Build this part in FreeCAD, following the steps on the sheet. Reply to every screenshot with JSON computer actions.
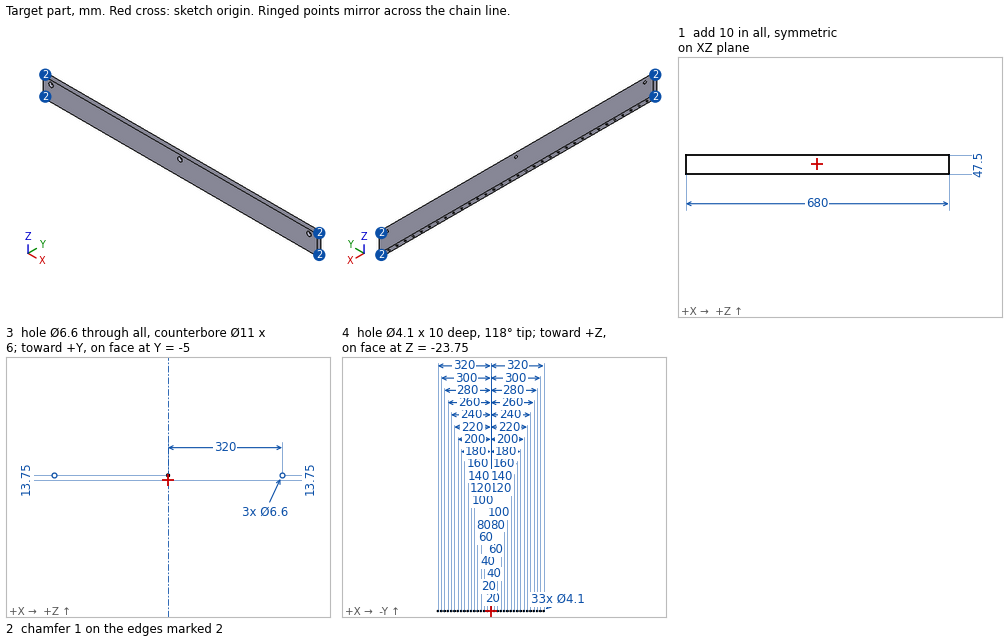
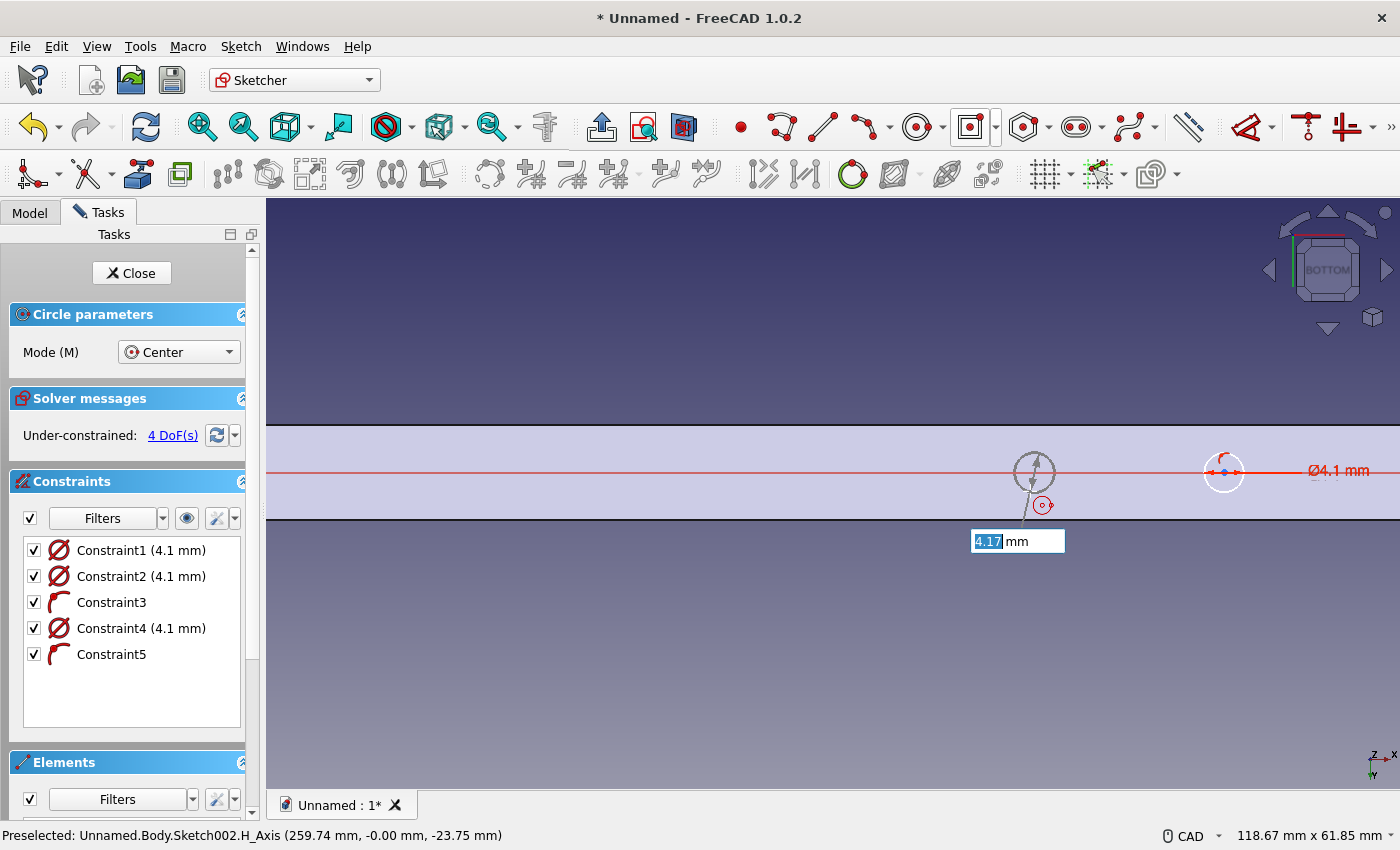
{"action": "type", "text": "4.1"}
{"action": "key", "text": "Return"}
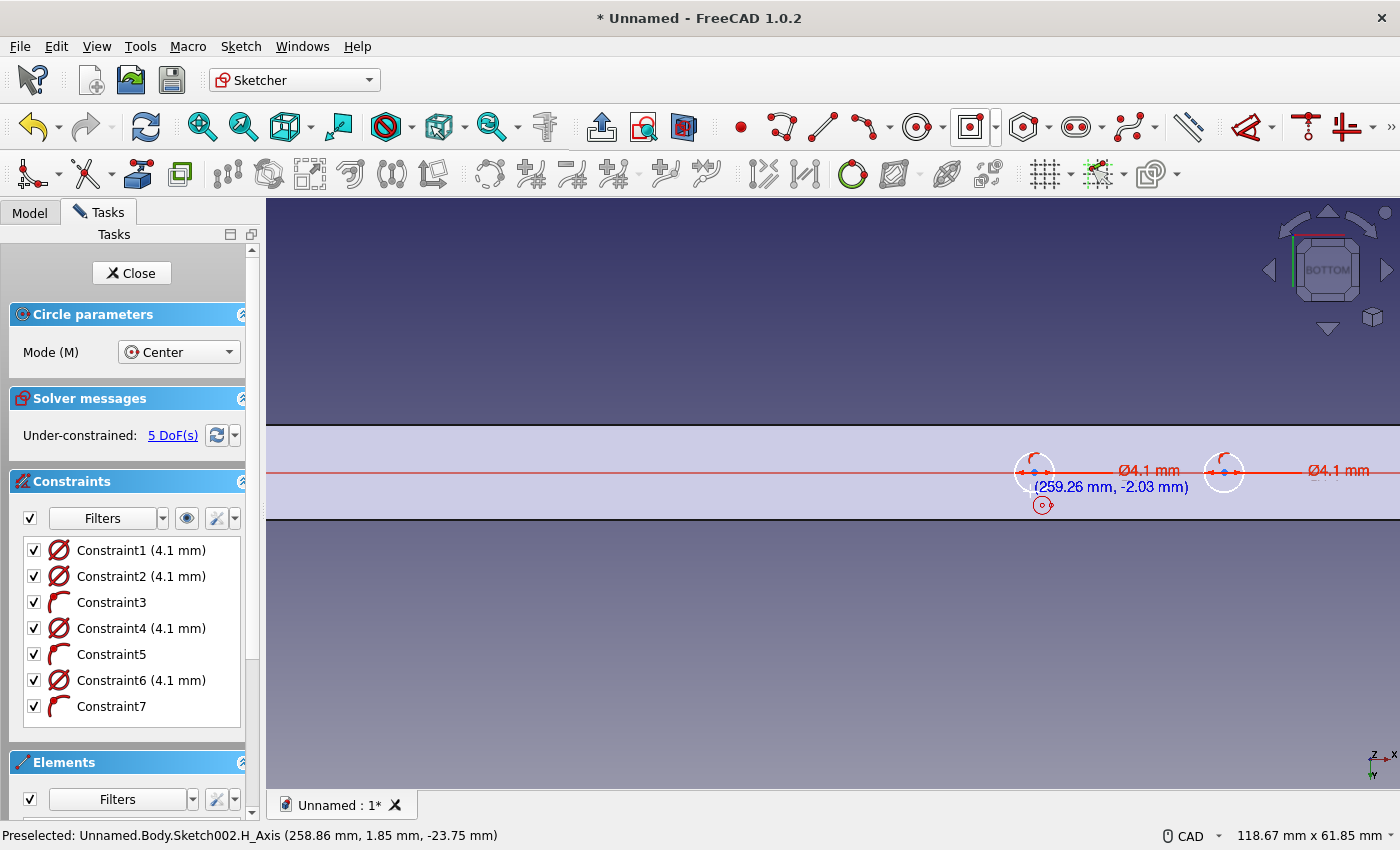
{"action": "scroll", "coordinate": [1040, 496], "scroll_direction": "down", "scroll_amount": 11}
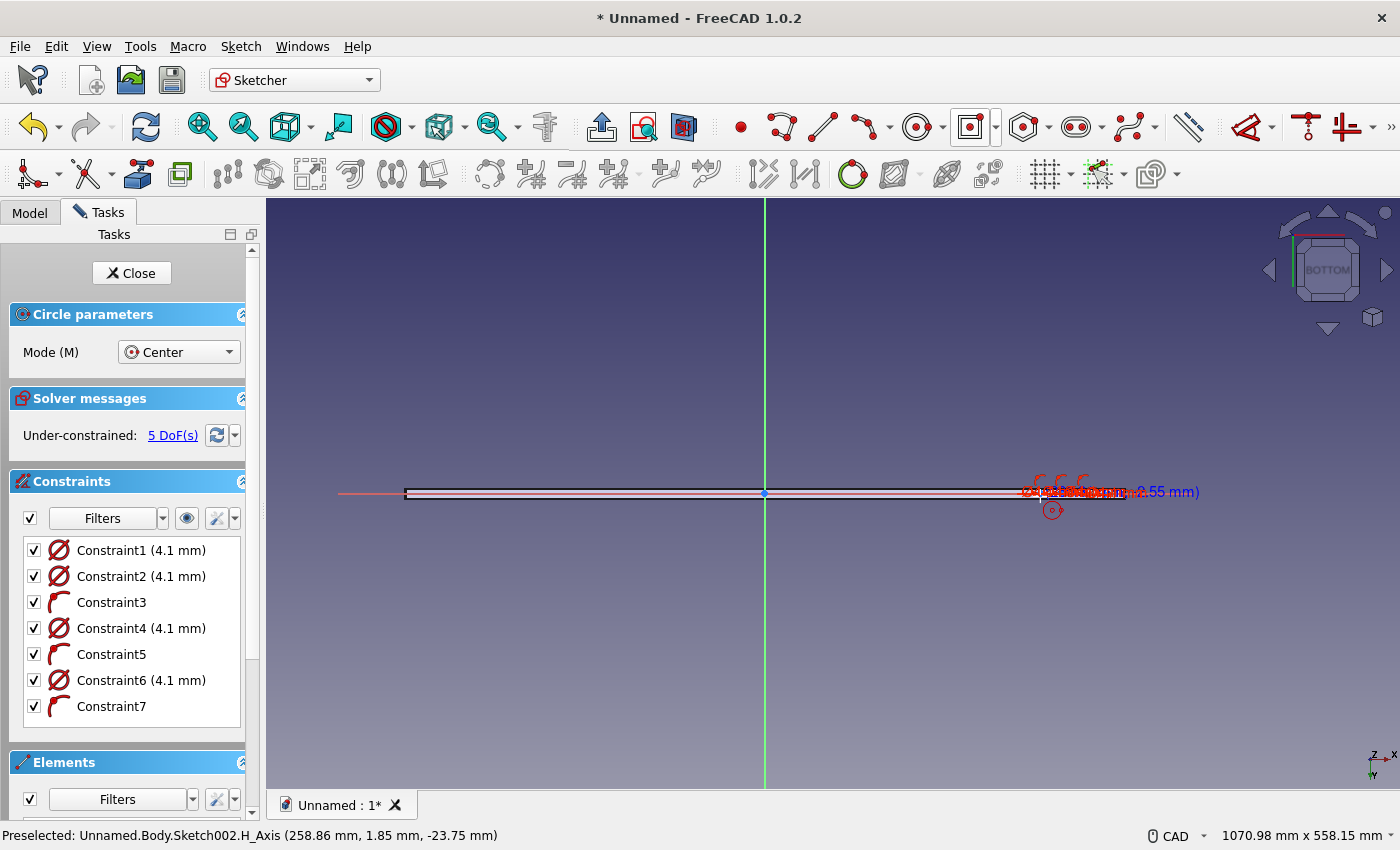
{"action": "left_click", "coordinate": [1019, 494]}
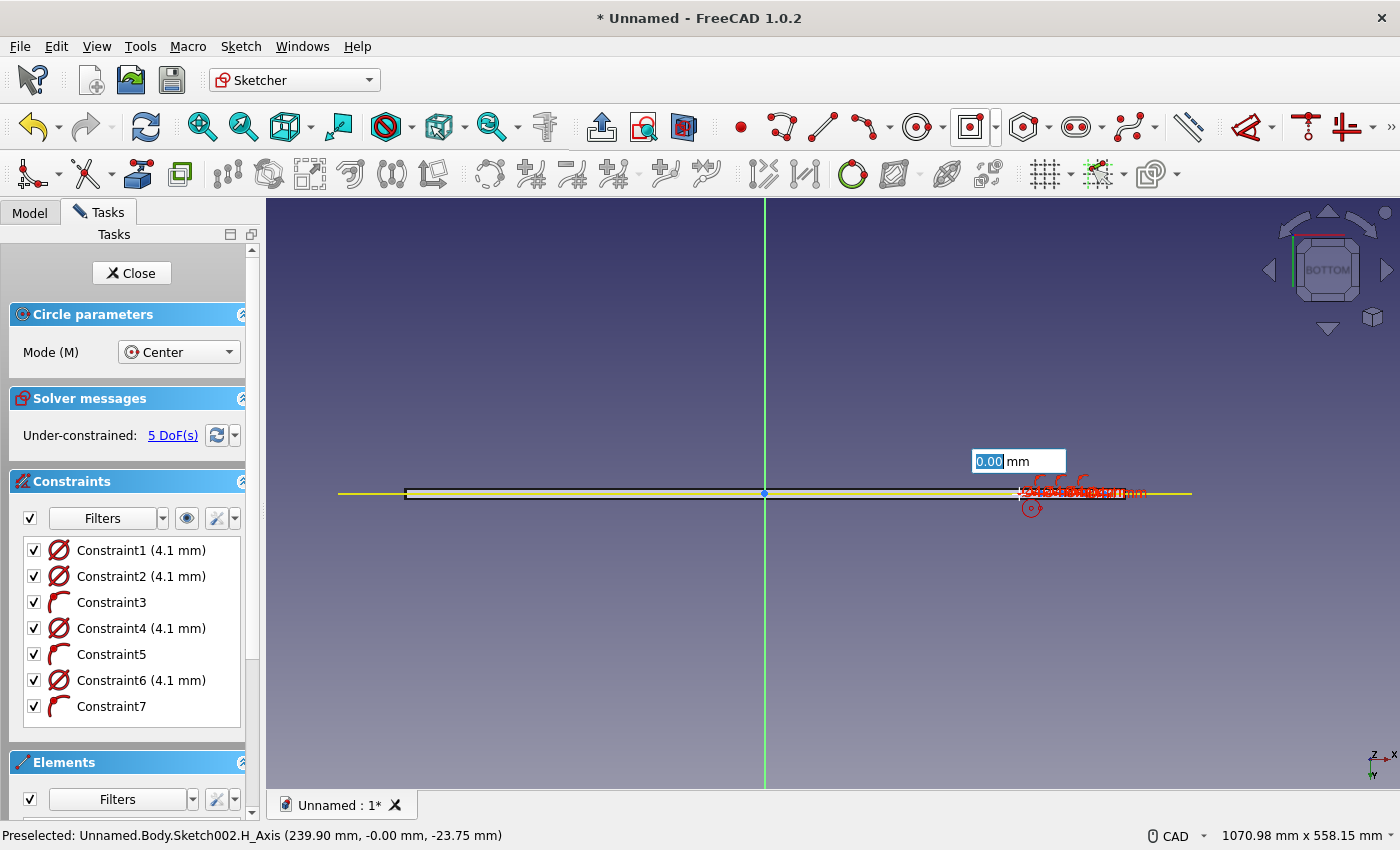
{"action": "scroll", "coordinate": [1018, 496], "scroll_direction": "up", "scroll_amount": 11}
{"action": "mouse_move", "coordinate": [1016, 491]}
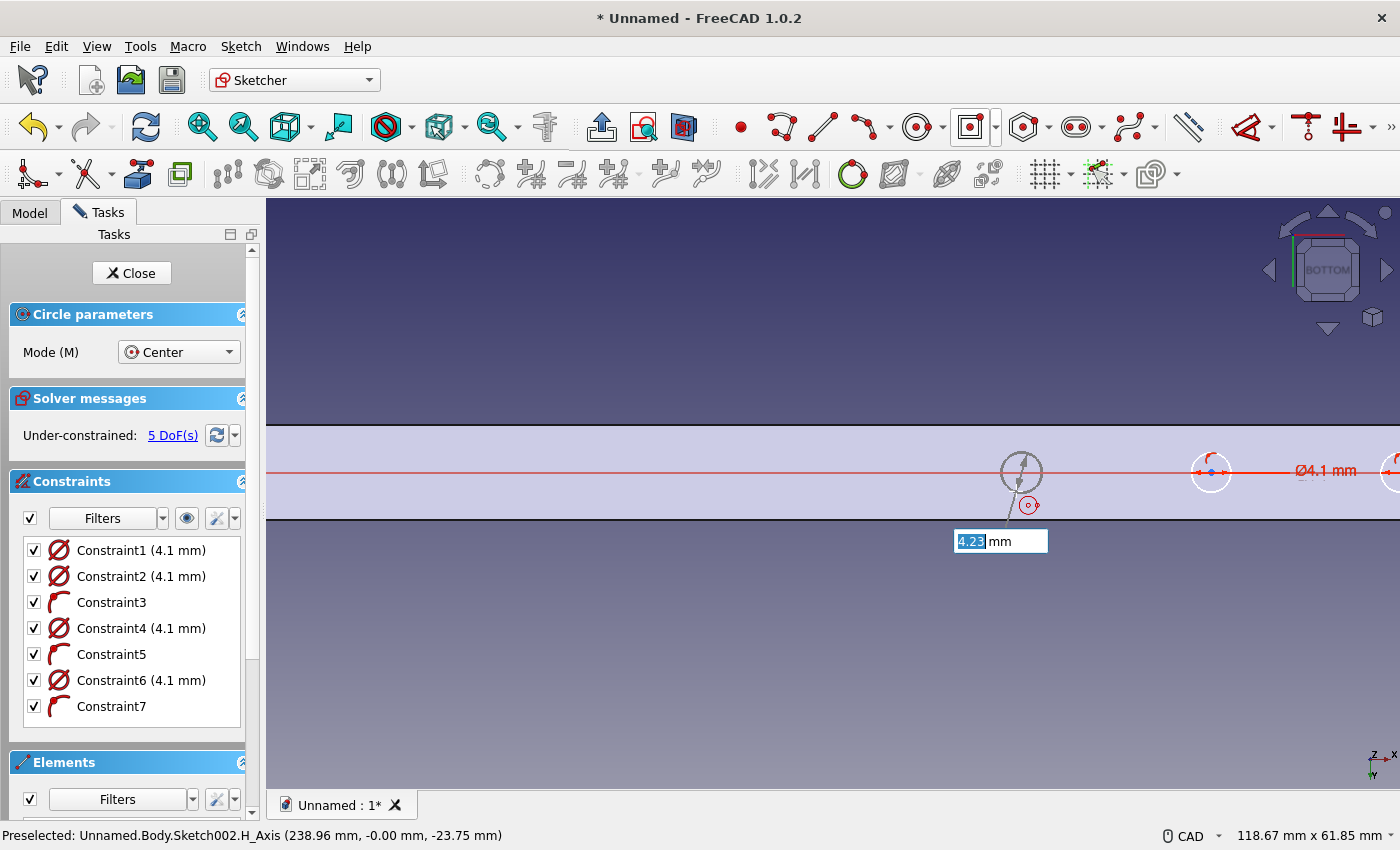
{"action": "type", "text": "4.1"}
{"action": "key", "text": "Return"}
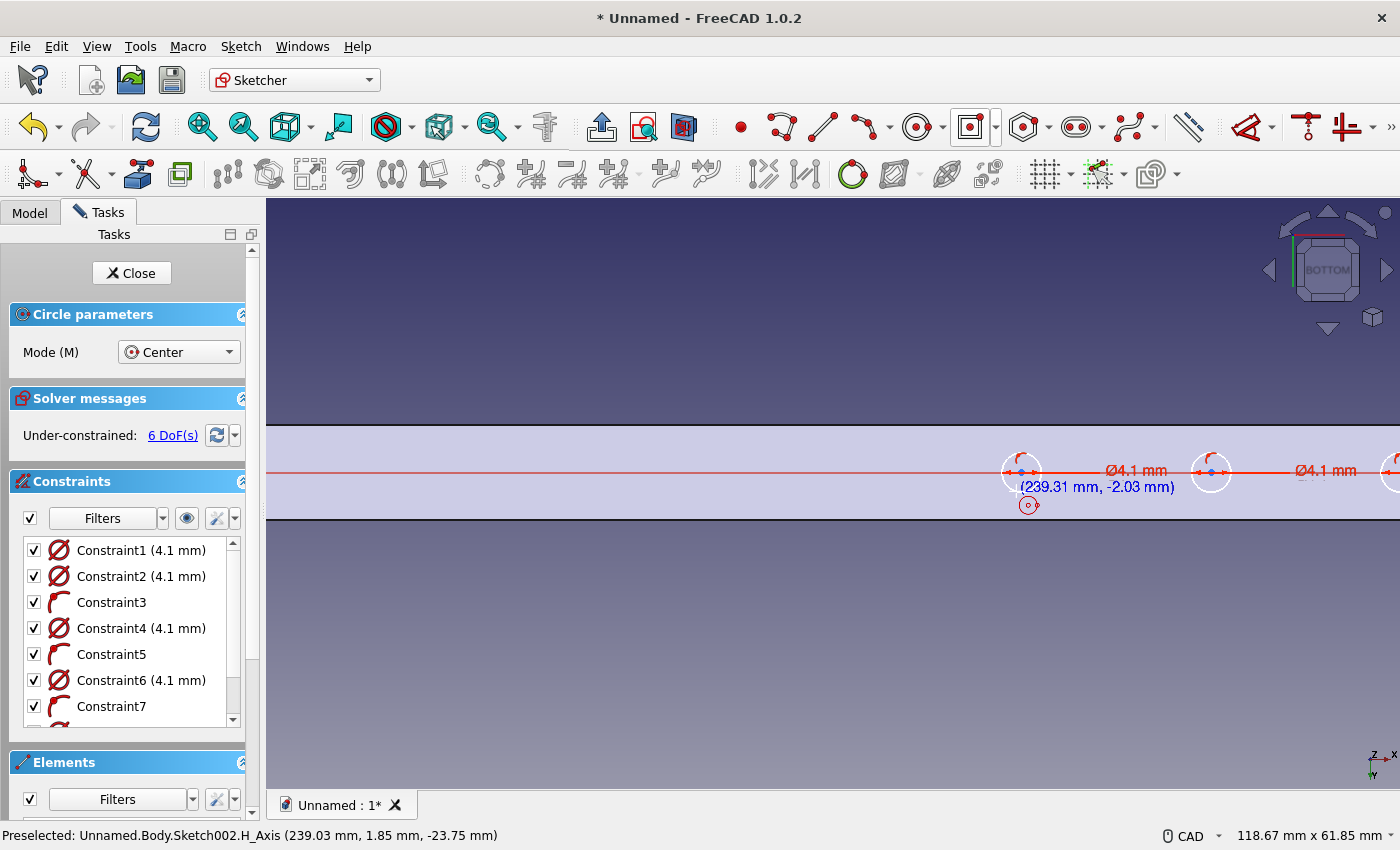
{"action": "scroll", "coordinate": [1018, 496], "scroll_direction": "down", "scroll_amount": 11}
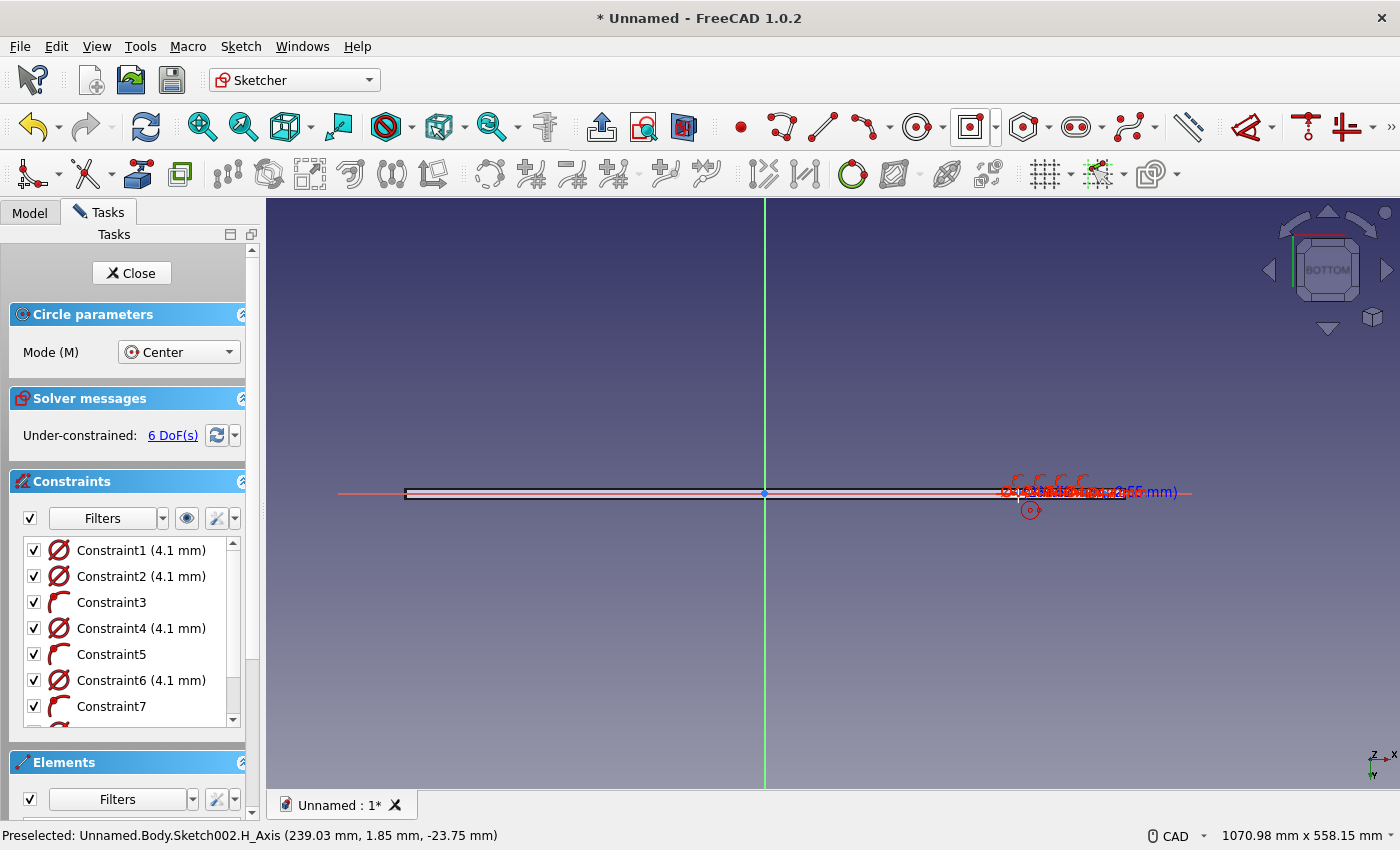
{"action": "left_click", "coordinate": [998, 494]}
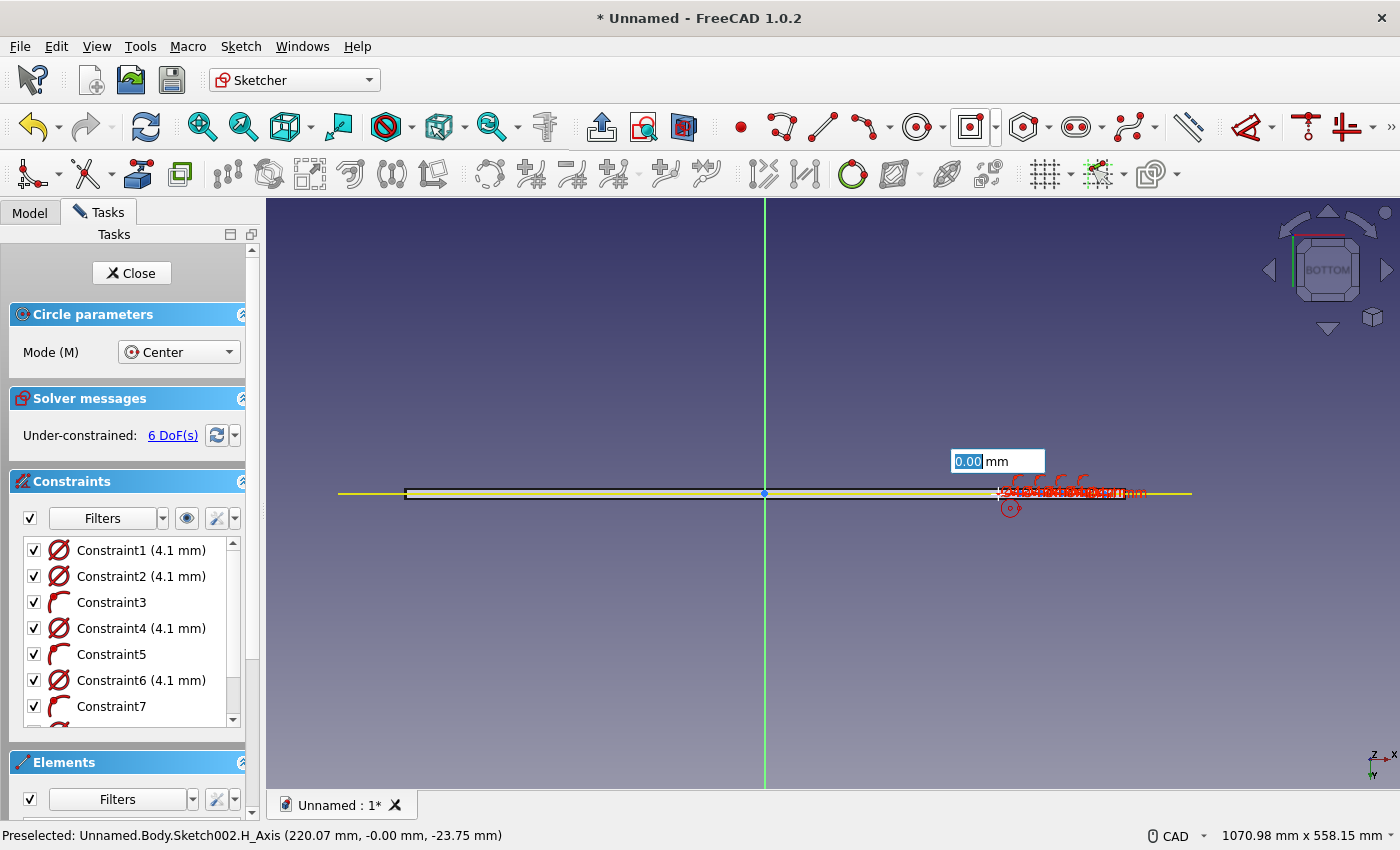
{"action": "scroll", "coordinate": [999, 492], "scroll_direction": "up", "scroll_amount": 11}
{"action": "mouse_move", "coordinate": [991, 486]}